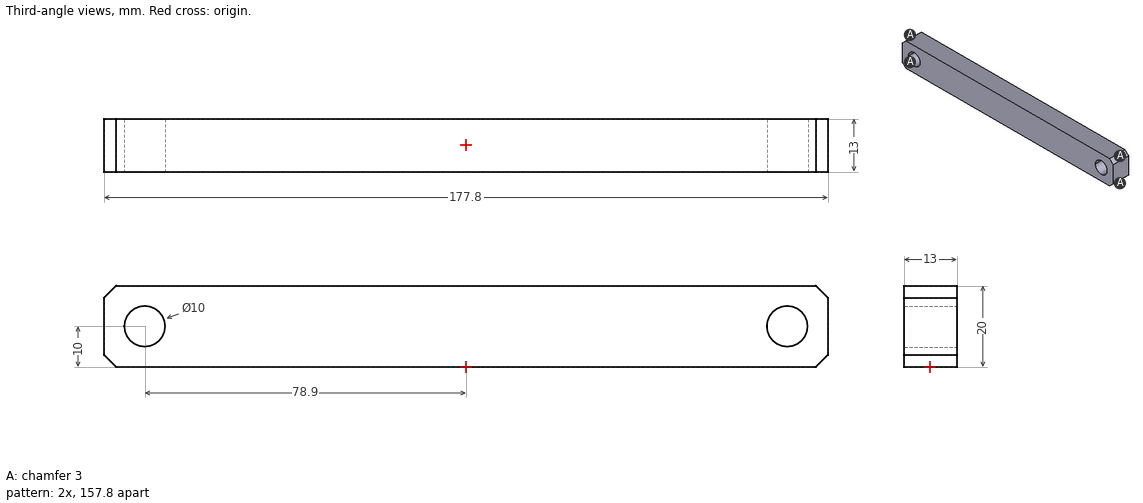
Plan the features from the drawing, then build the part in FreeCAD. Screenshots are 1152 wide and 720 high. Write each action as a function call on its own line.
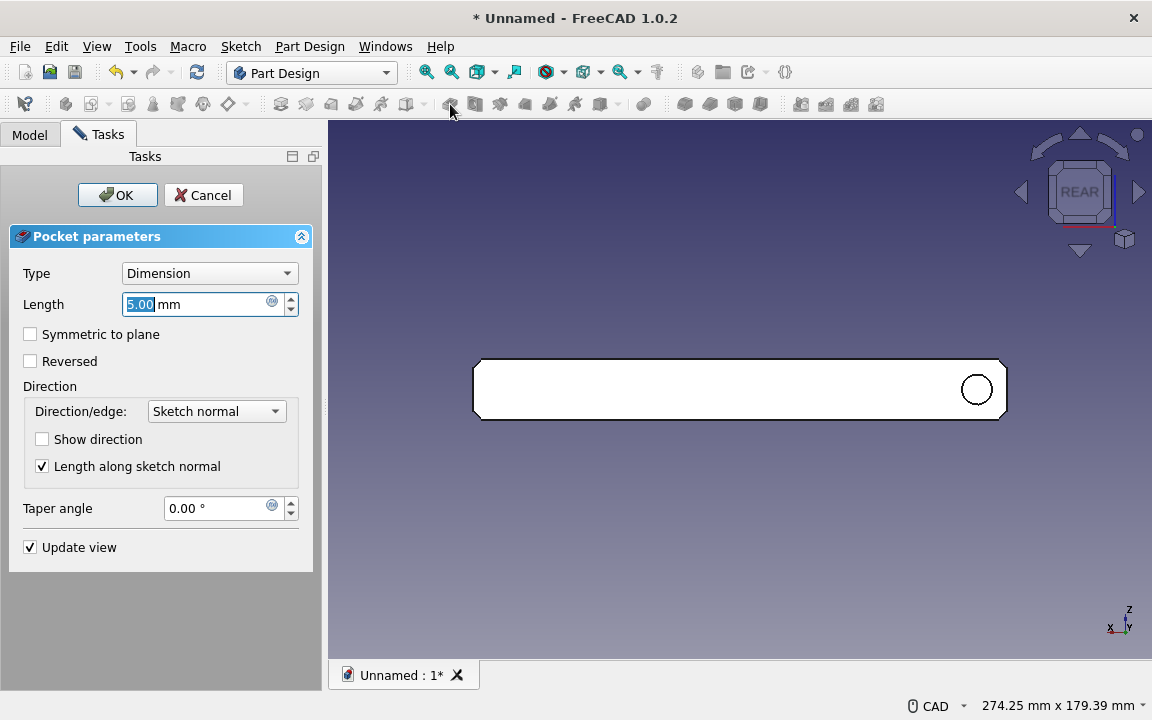
text(13)
key(Tab)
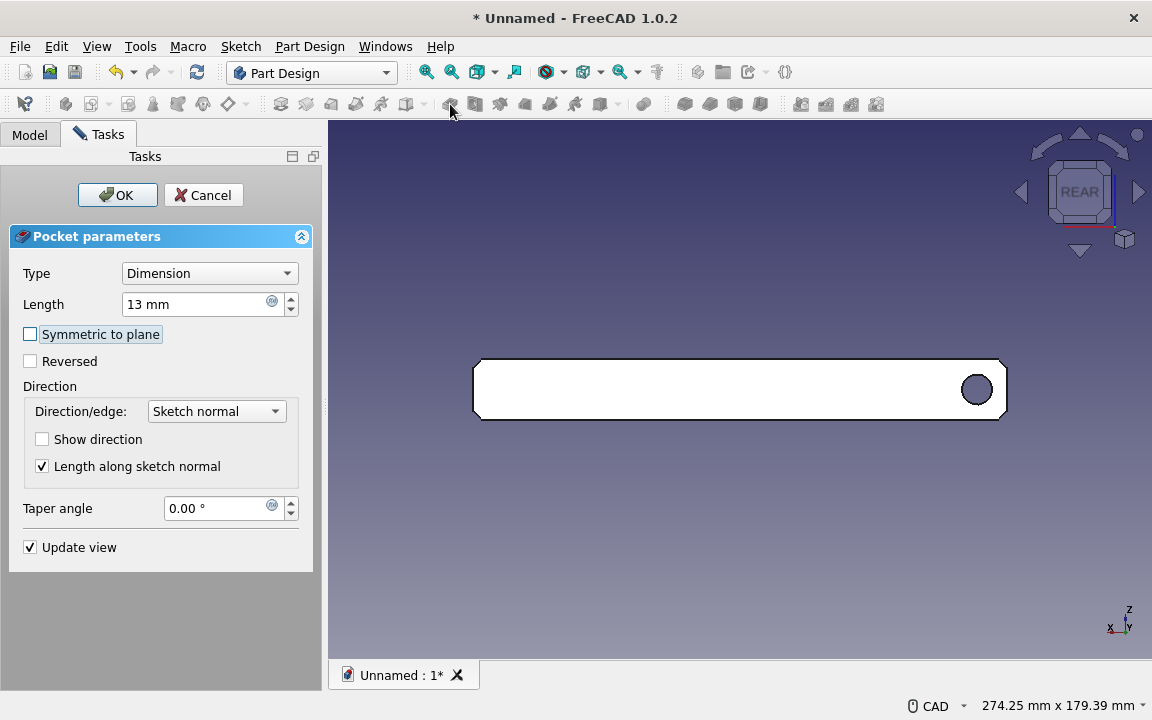
click(118, 195)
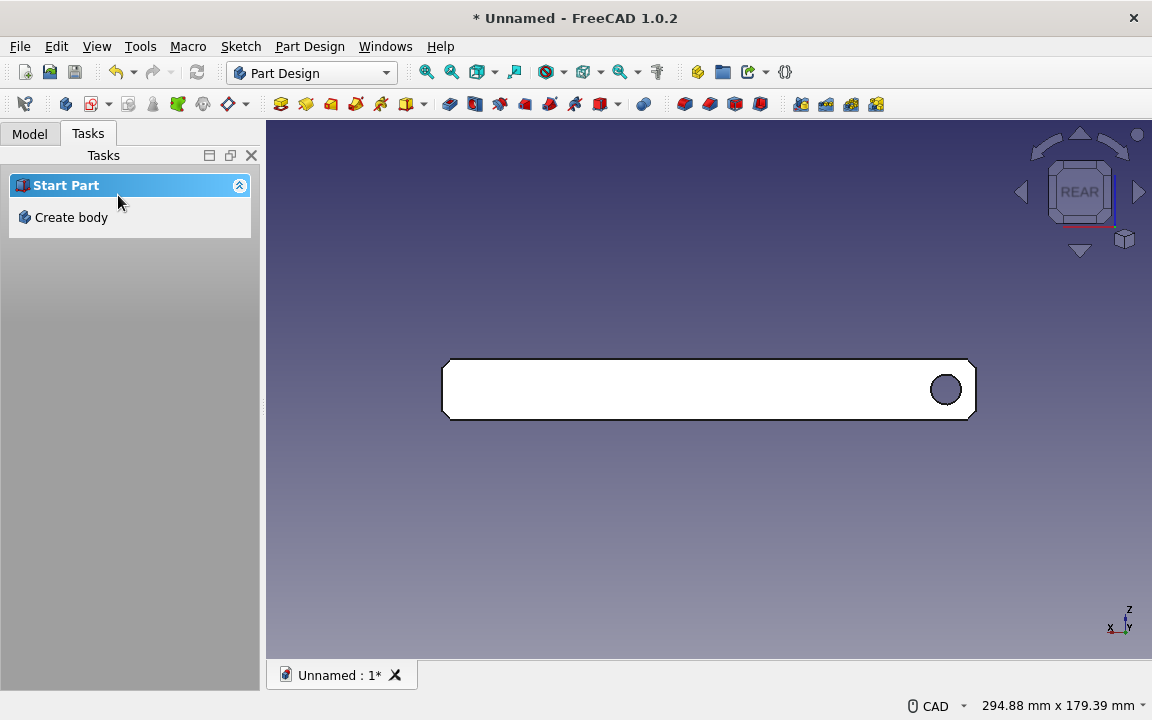
click(30, 134)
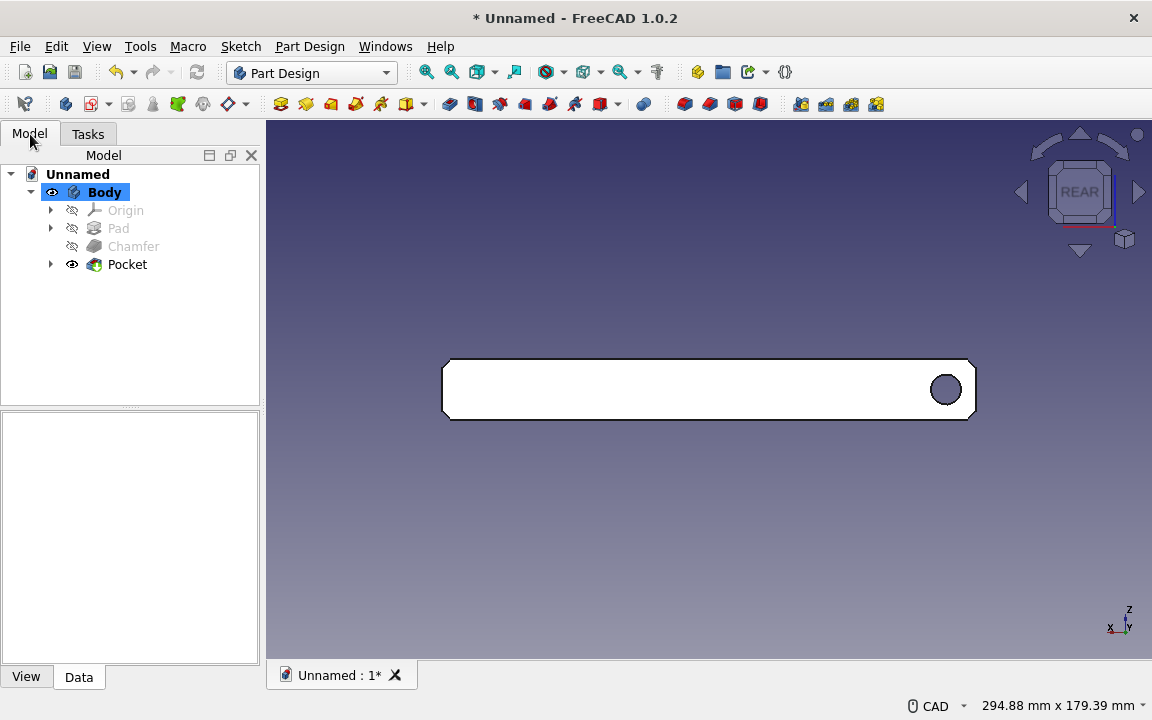
click(117, 264)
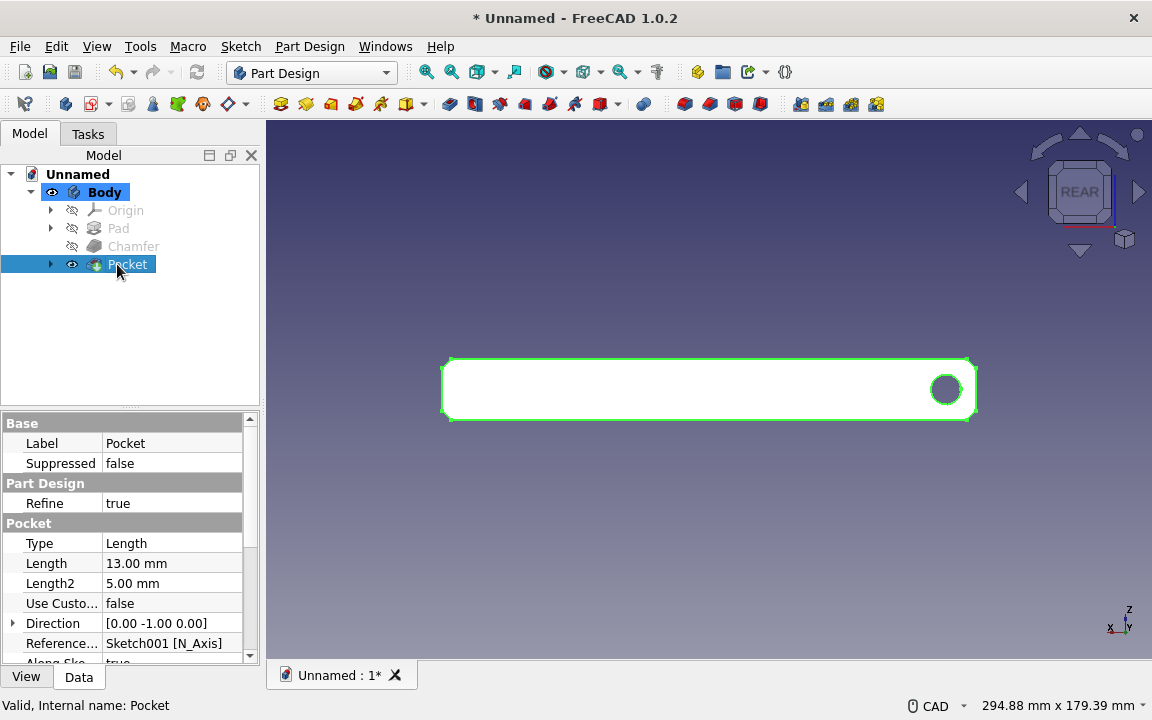
click(826, 104)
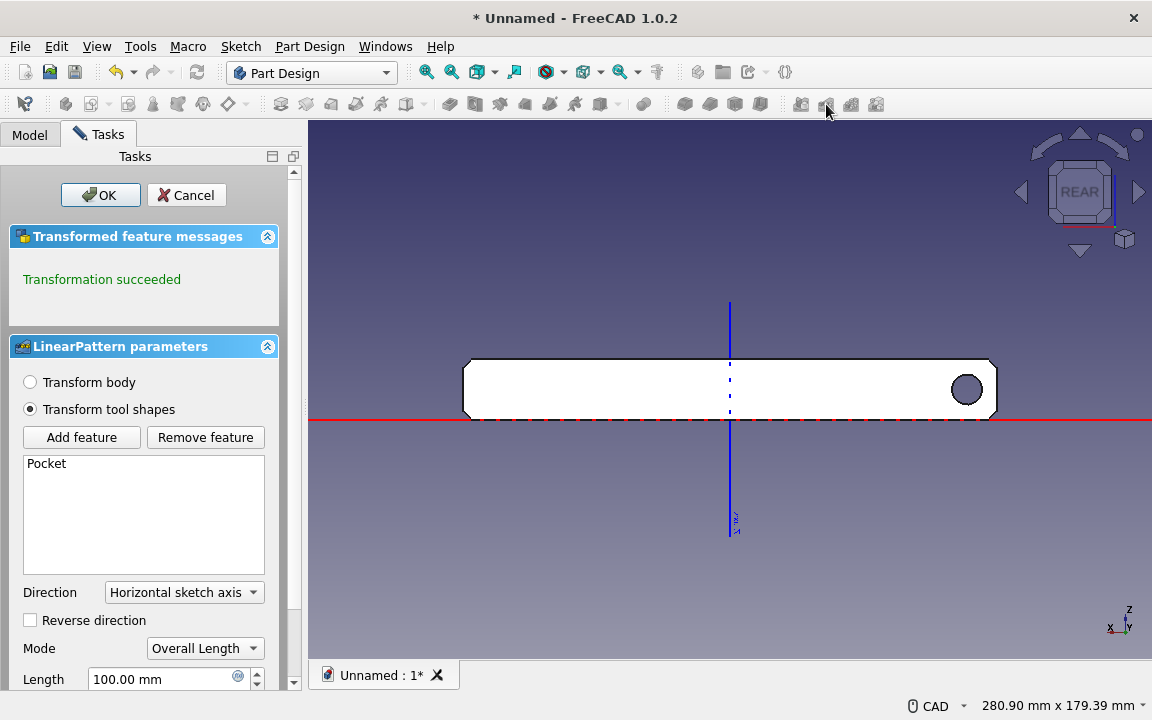
click(185, 592)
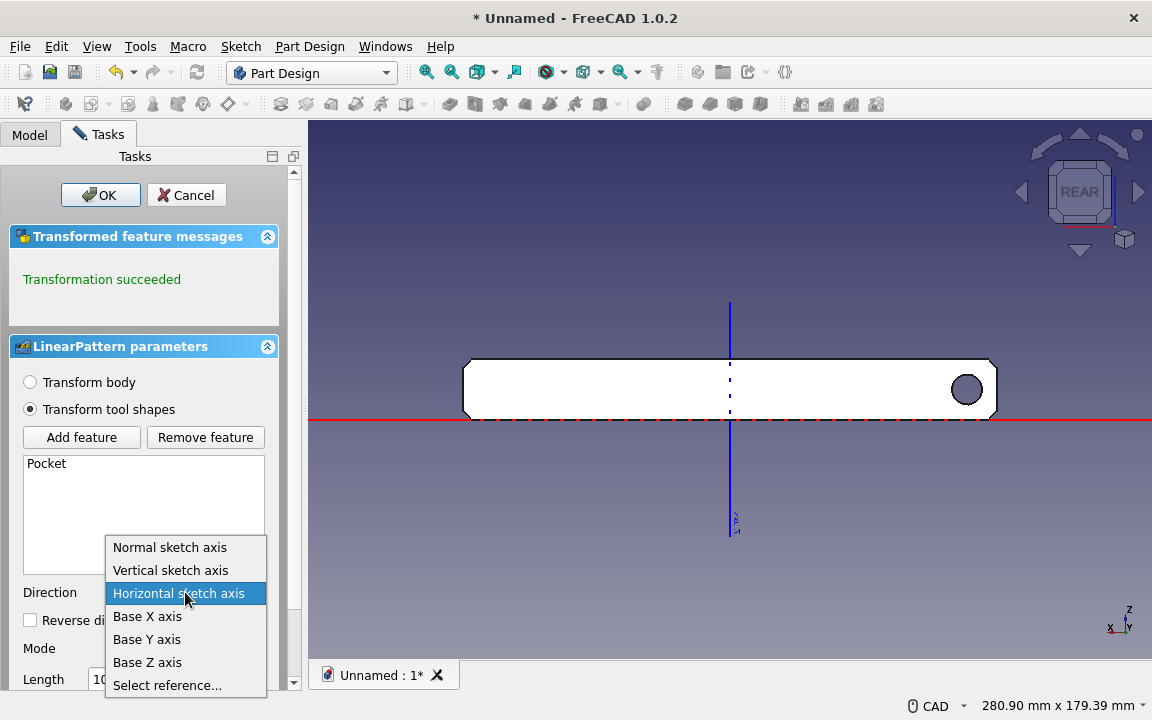
click(184, 616)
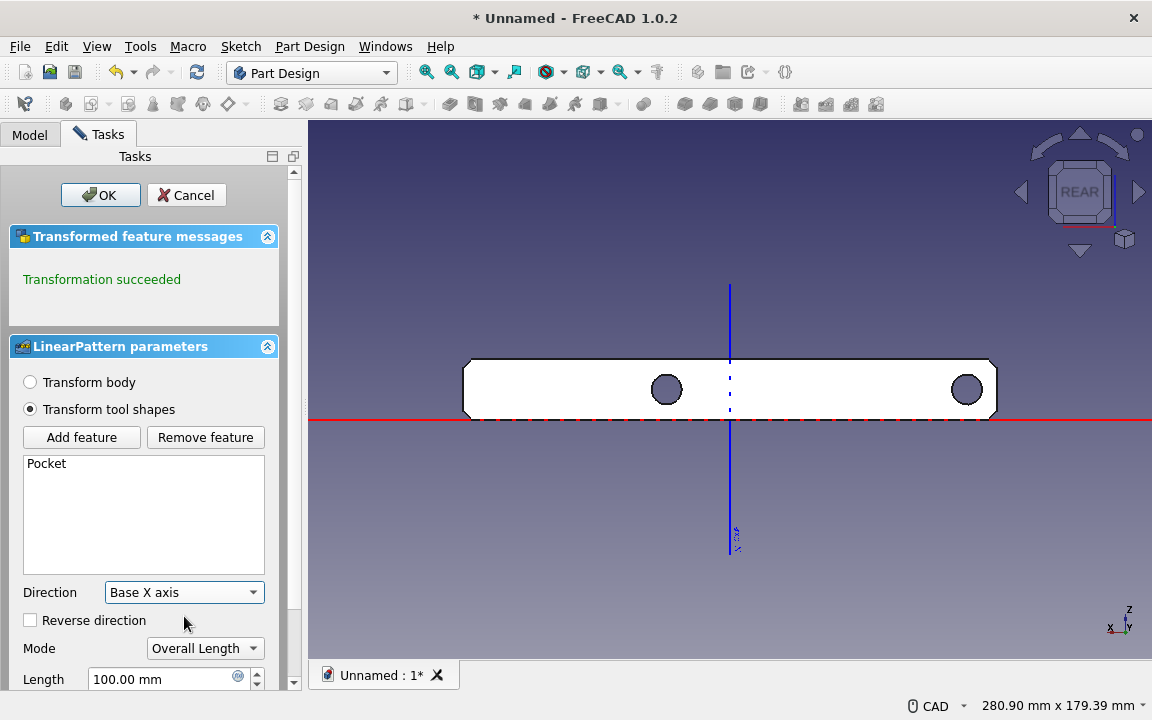
click(206, 648)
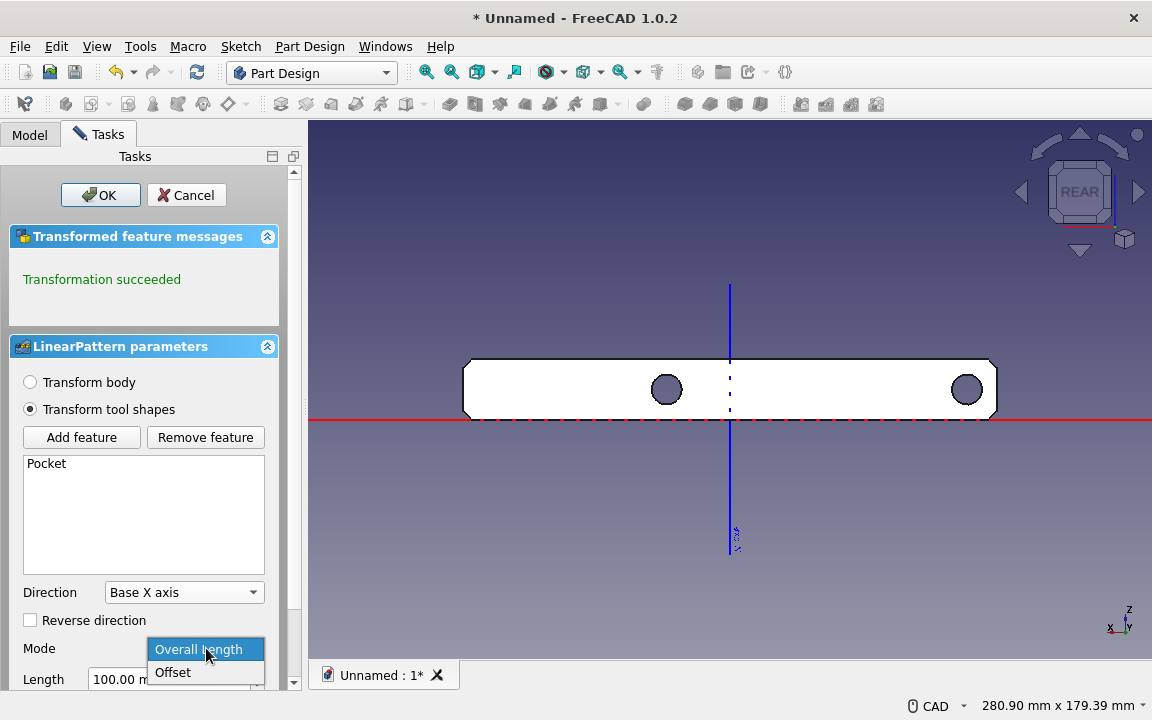
click(204, 672)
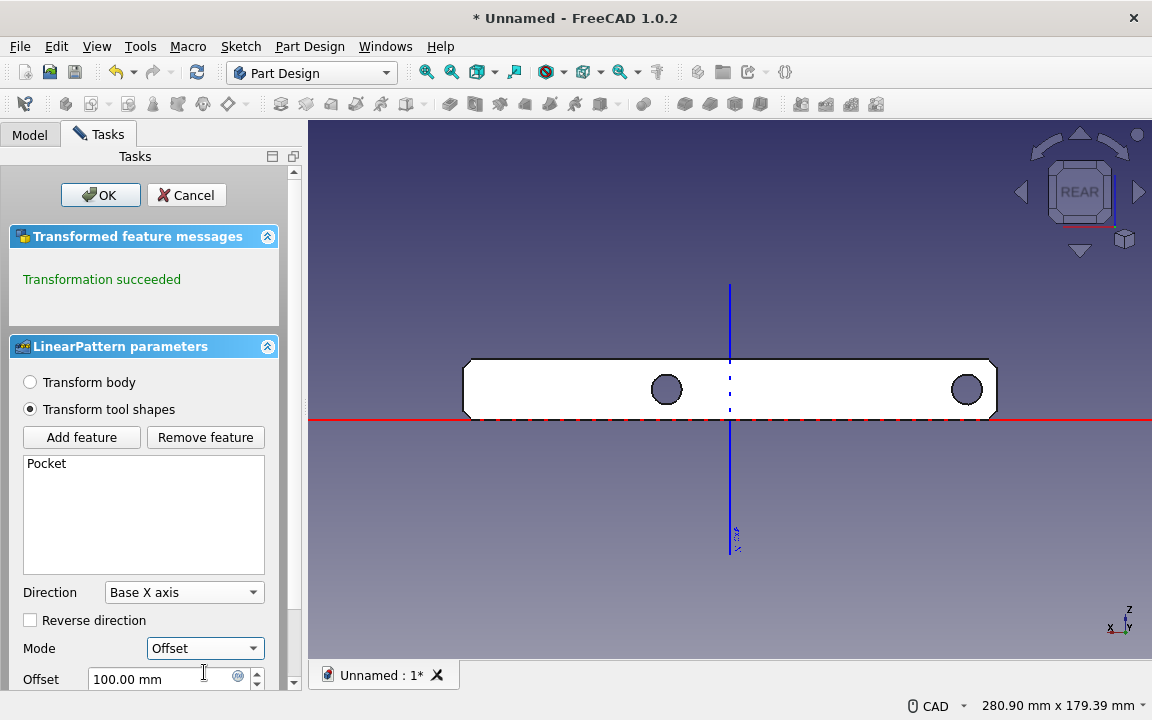
scroll(294, 428, down, 2)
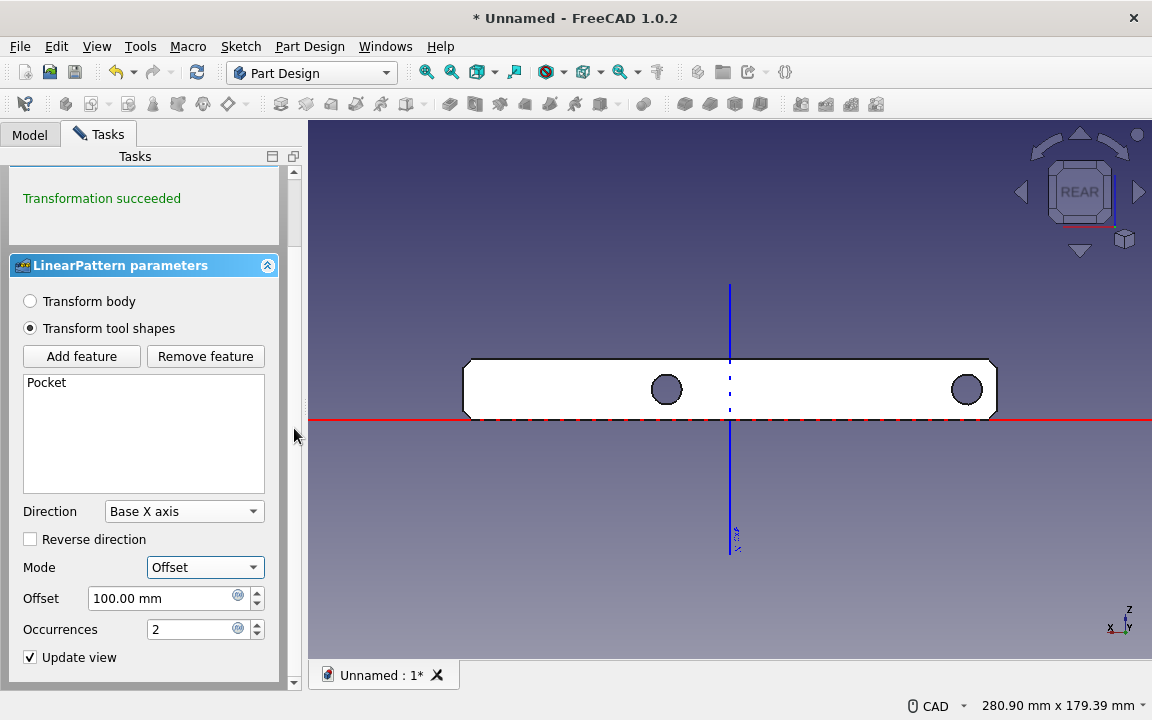
triple_click(170, 598)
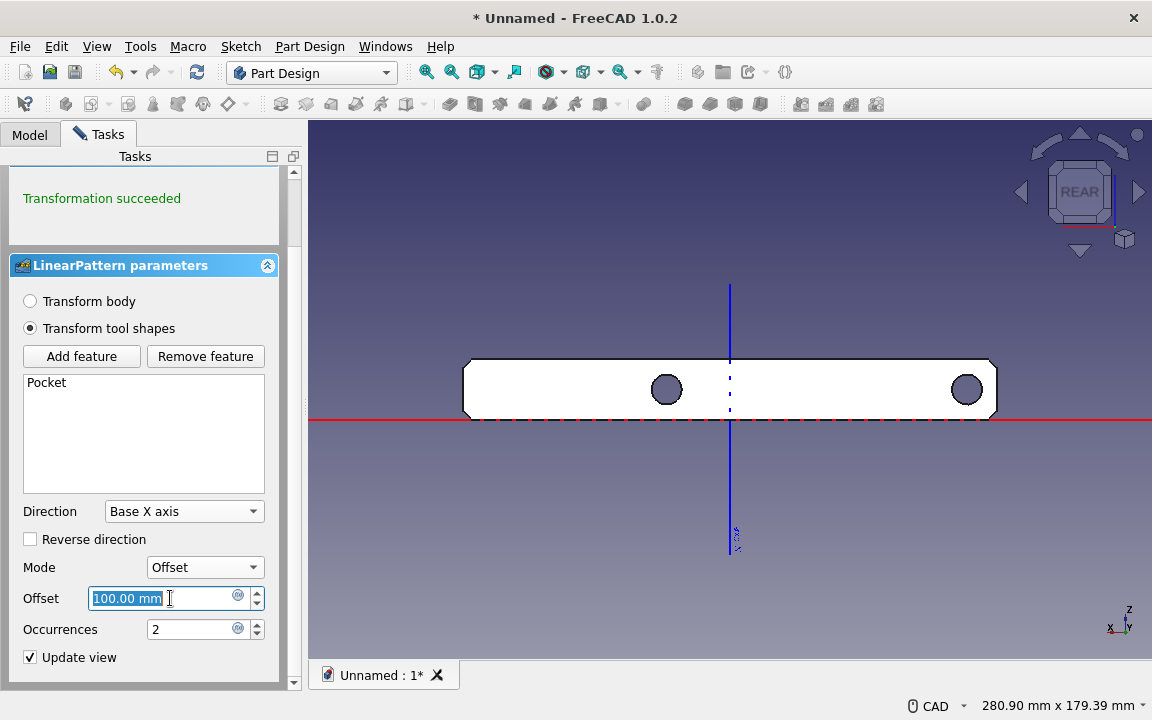
text(157.8)
key(Tab)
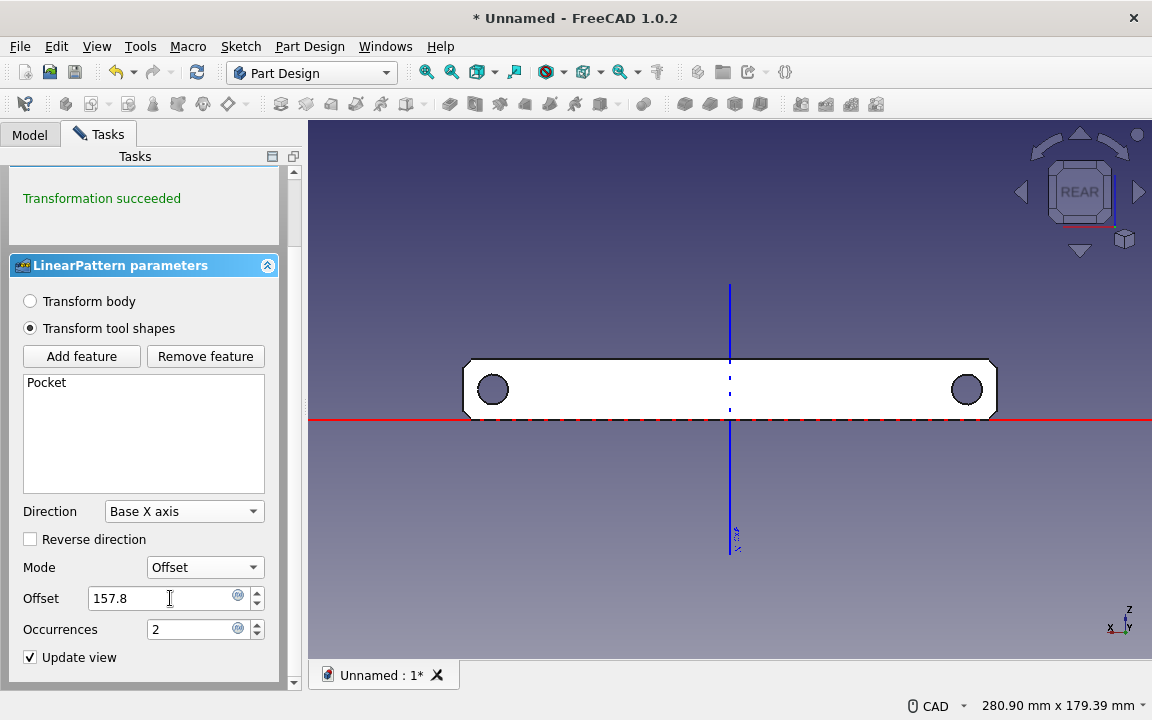
triple_click(199, 630)